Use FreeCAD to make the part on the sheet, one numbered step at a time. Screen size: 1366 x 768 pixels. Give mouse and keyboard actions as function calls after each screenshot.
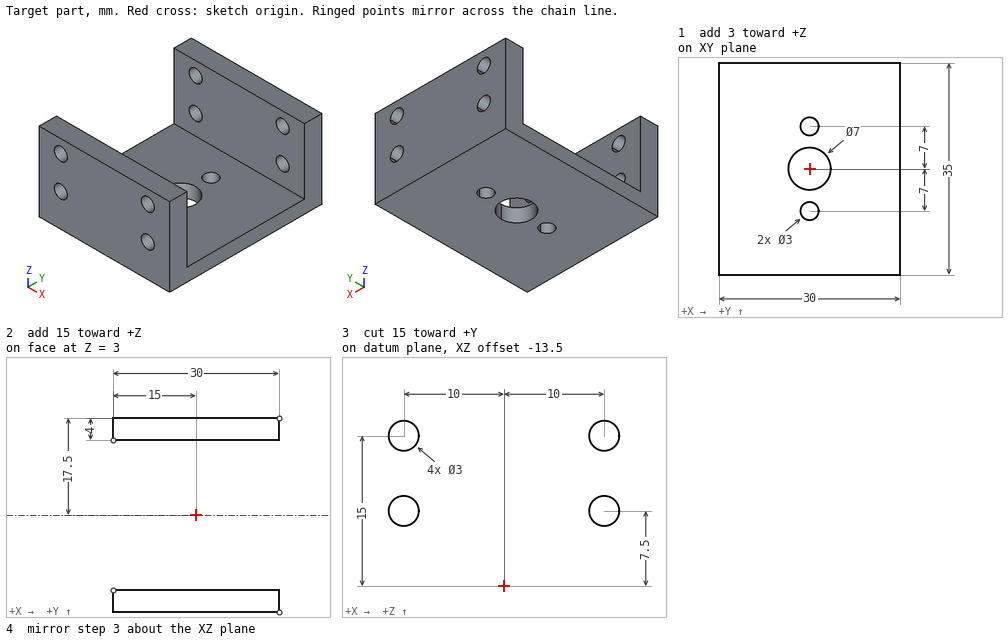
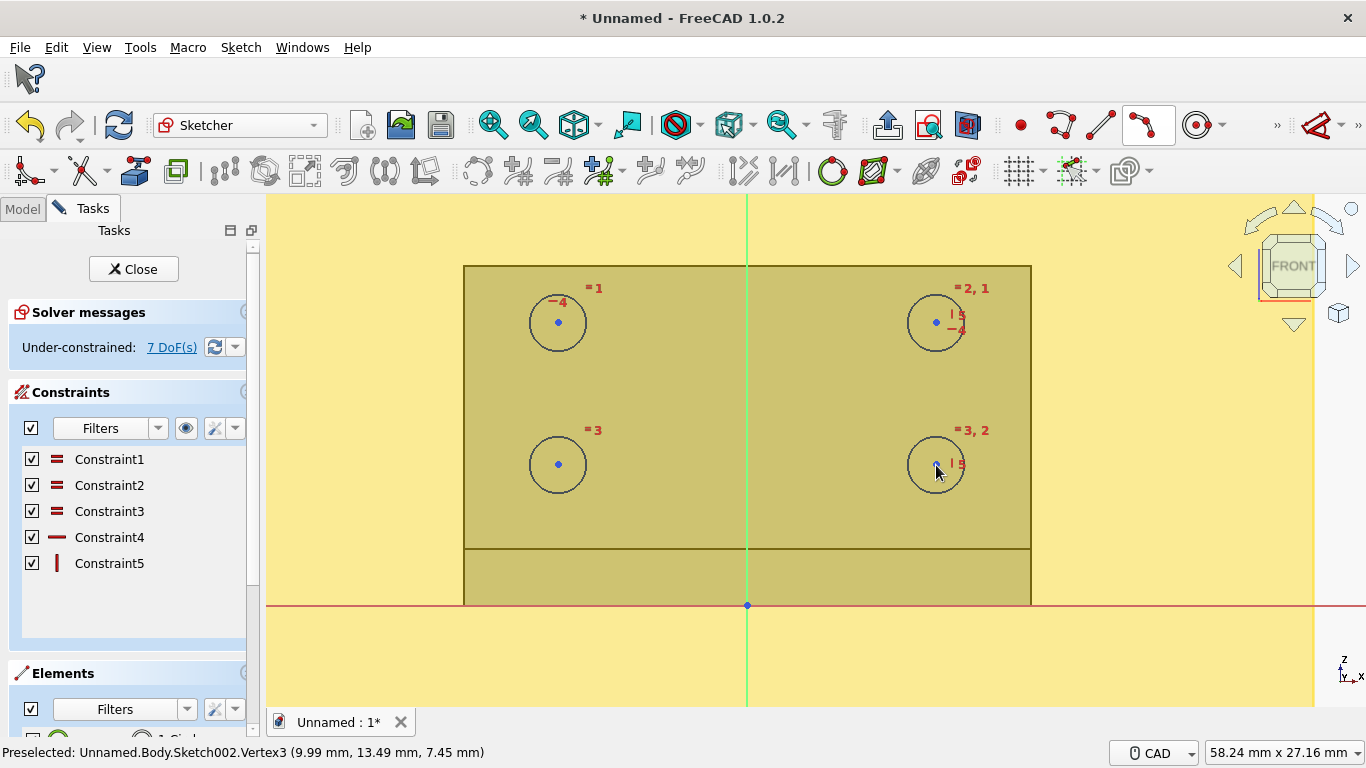
click(558, 323)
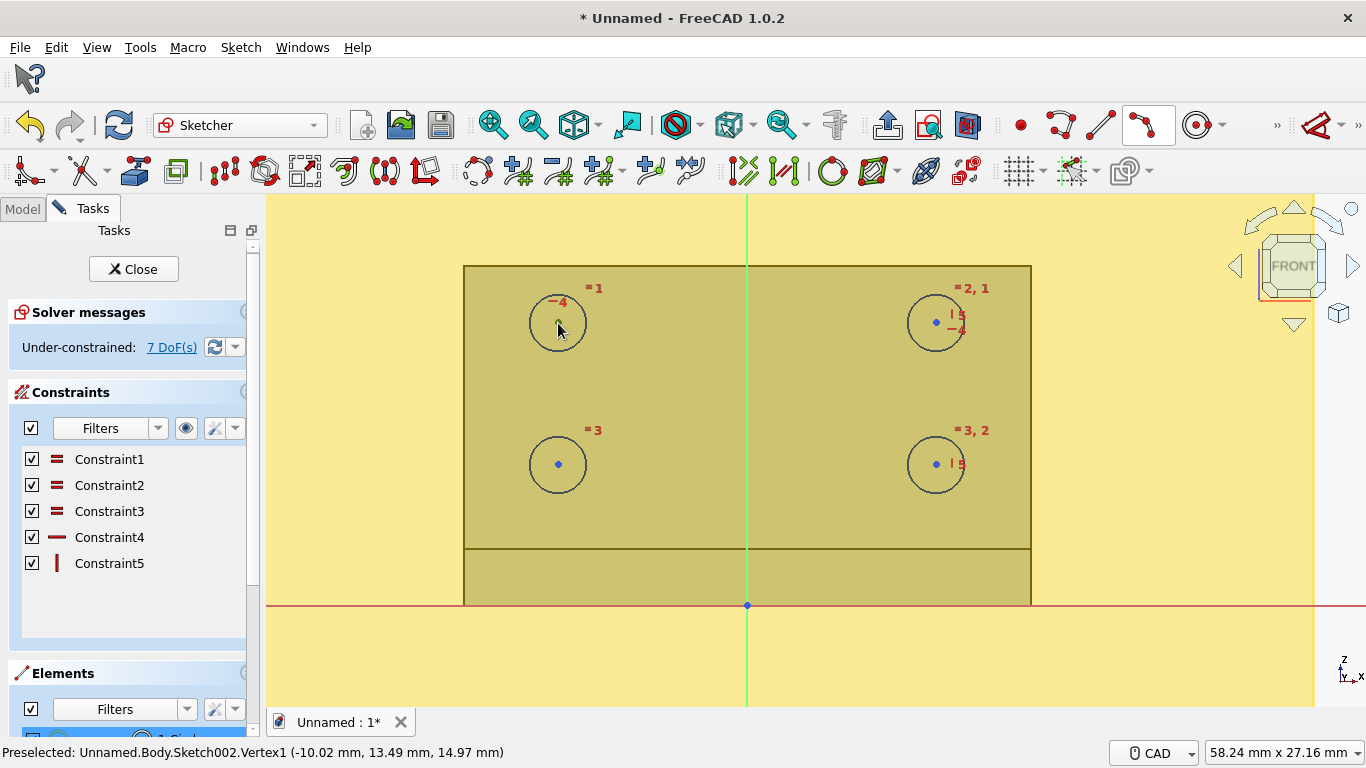
click(558, 465)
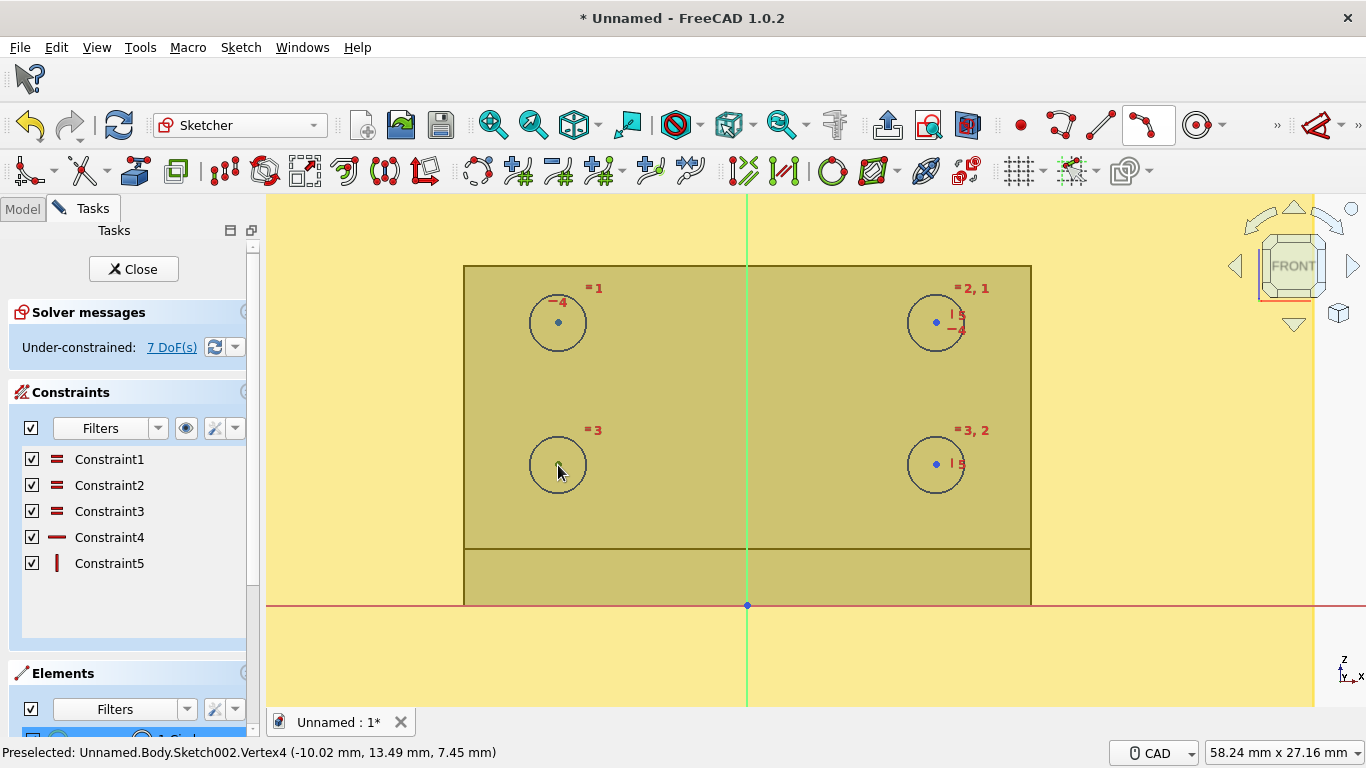
key(v)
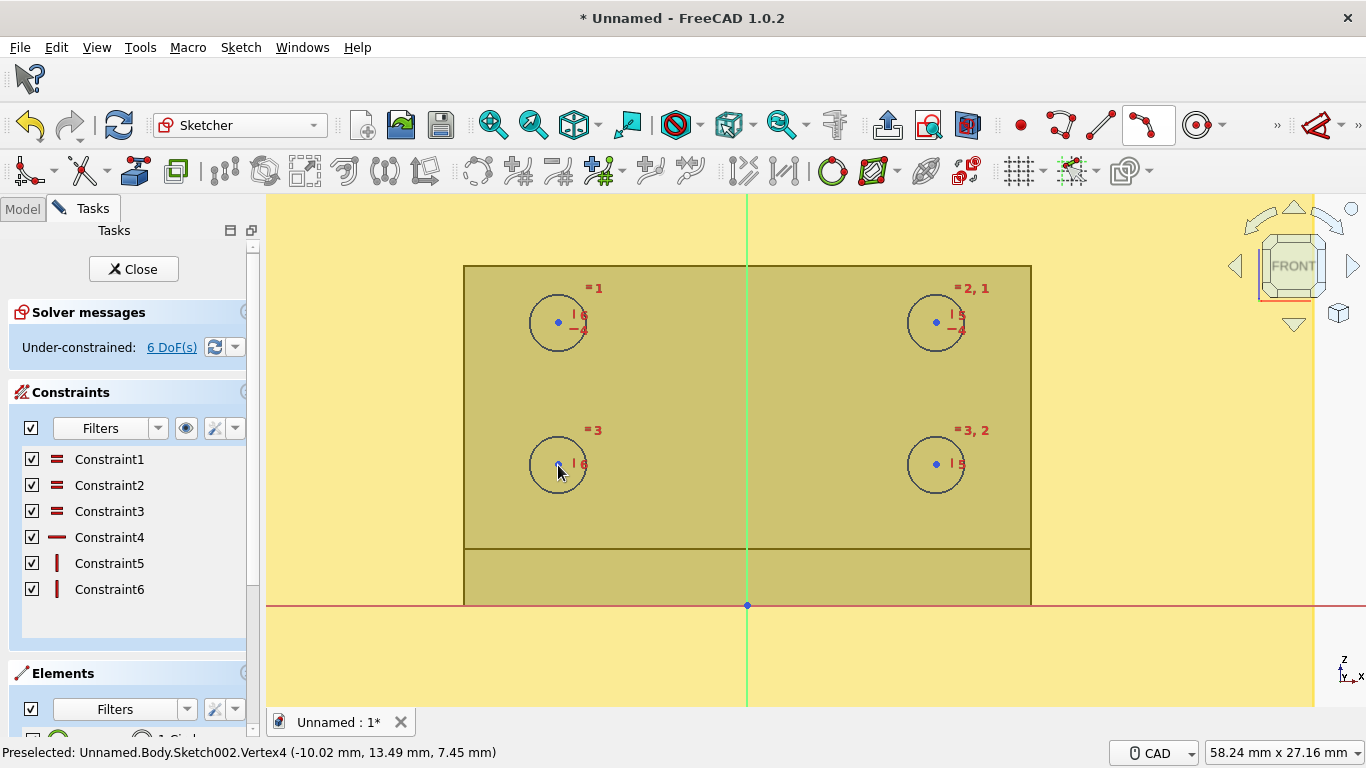
click(936, 465)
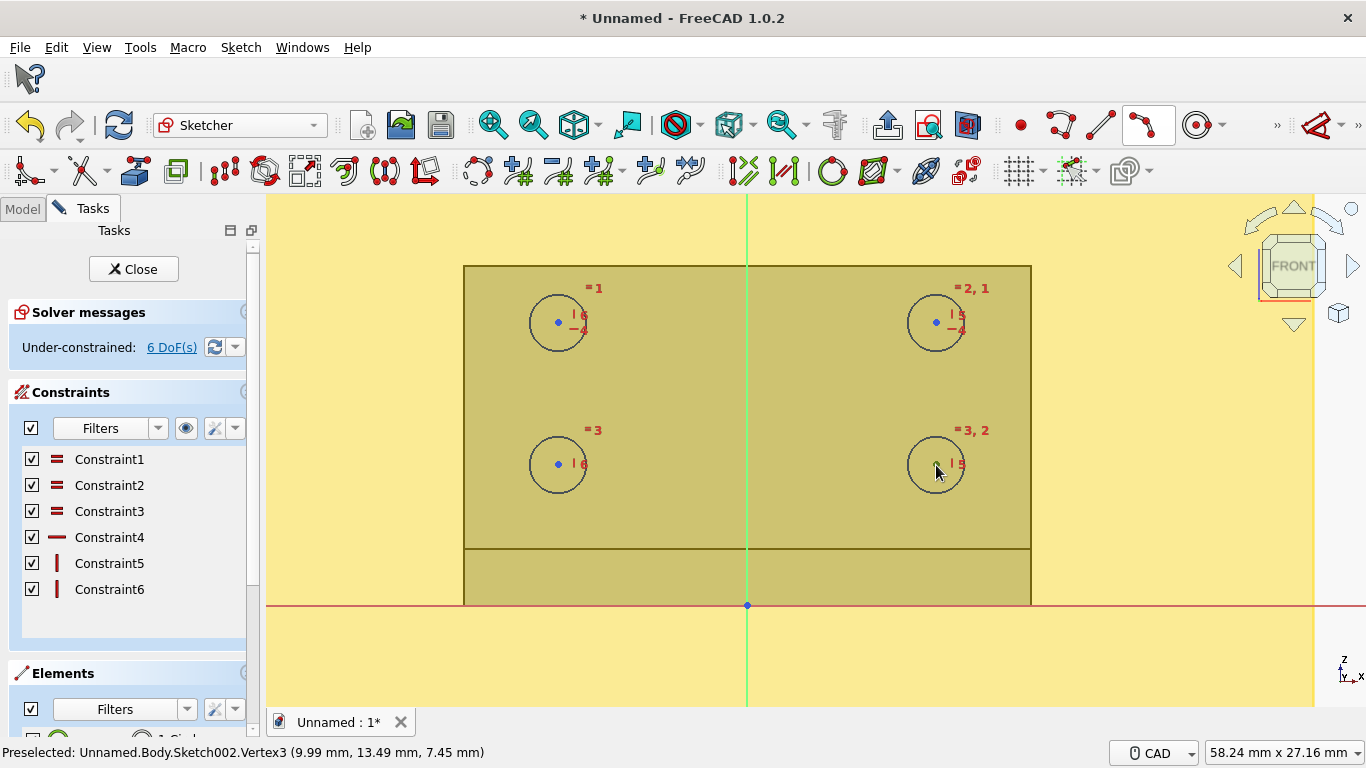
click(558, 465)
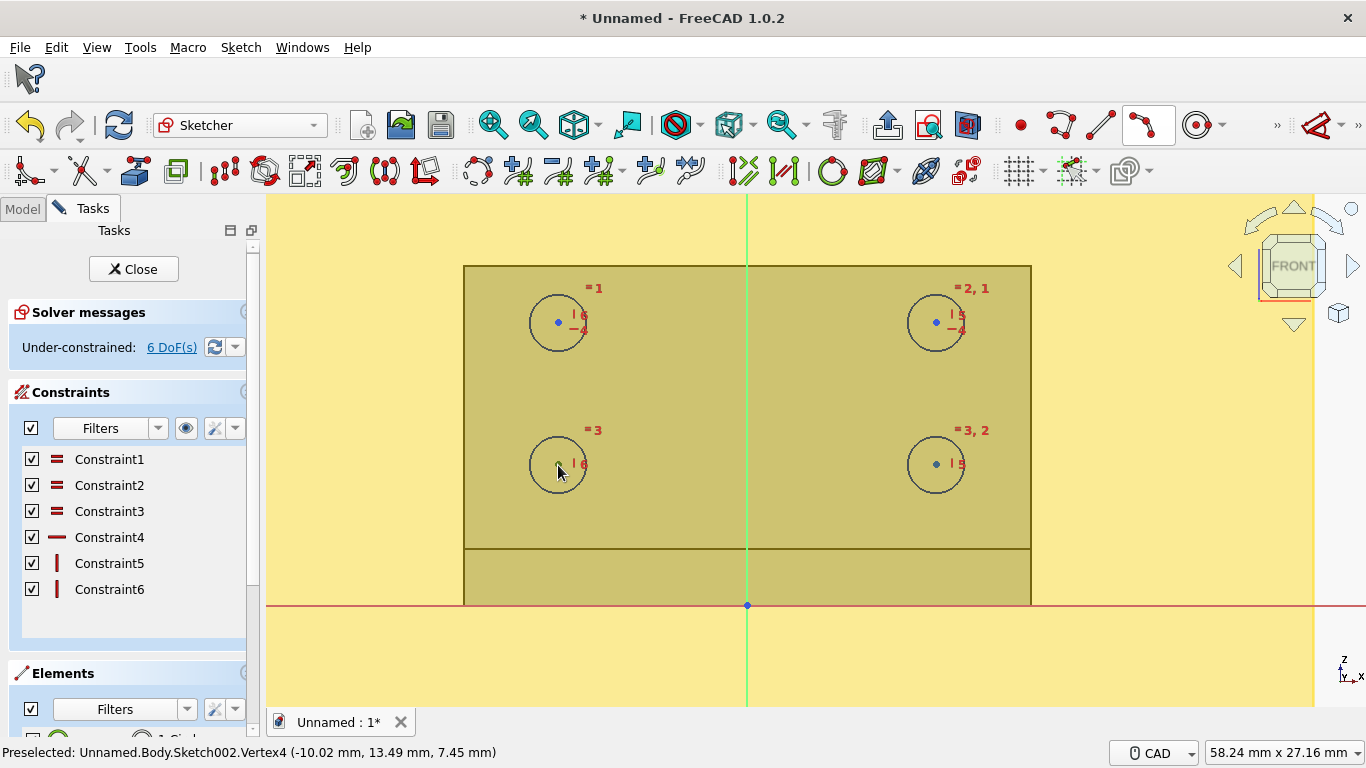
key(h)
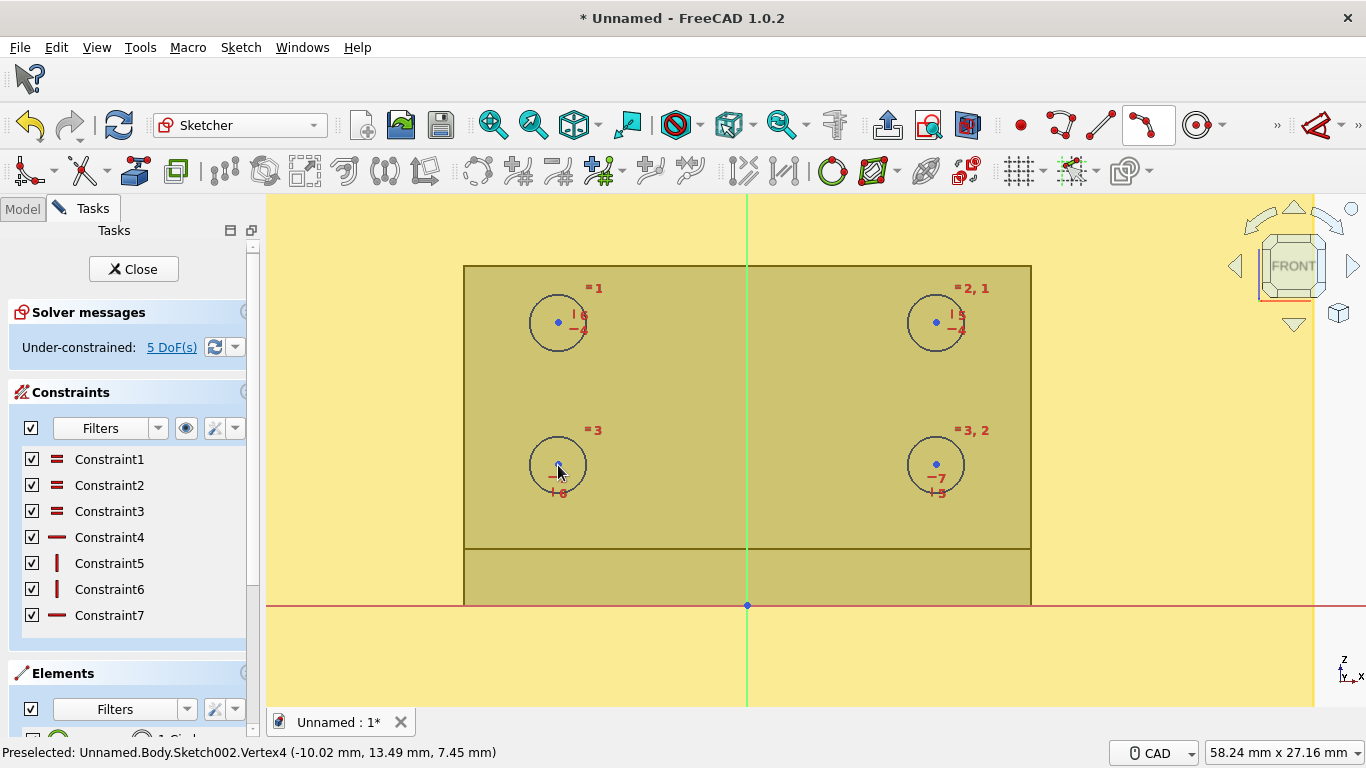
click(1316, 126)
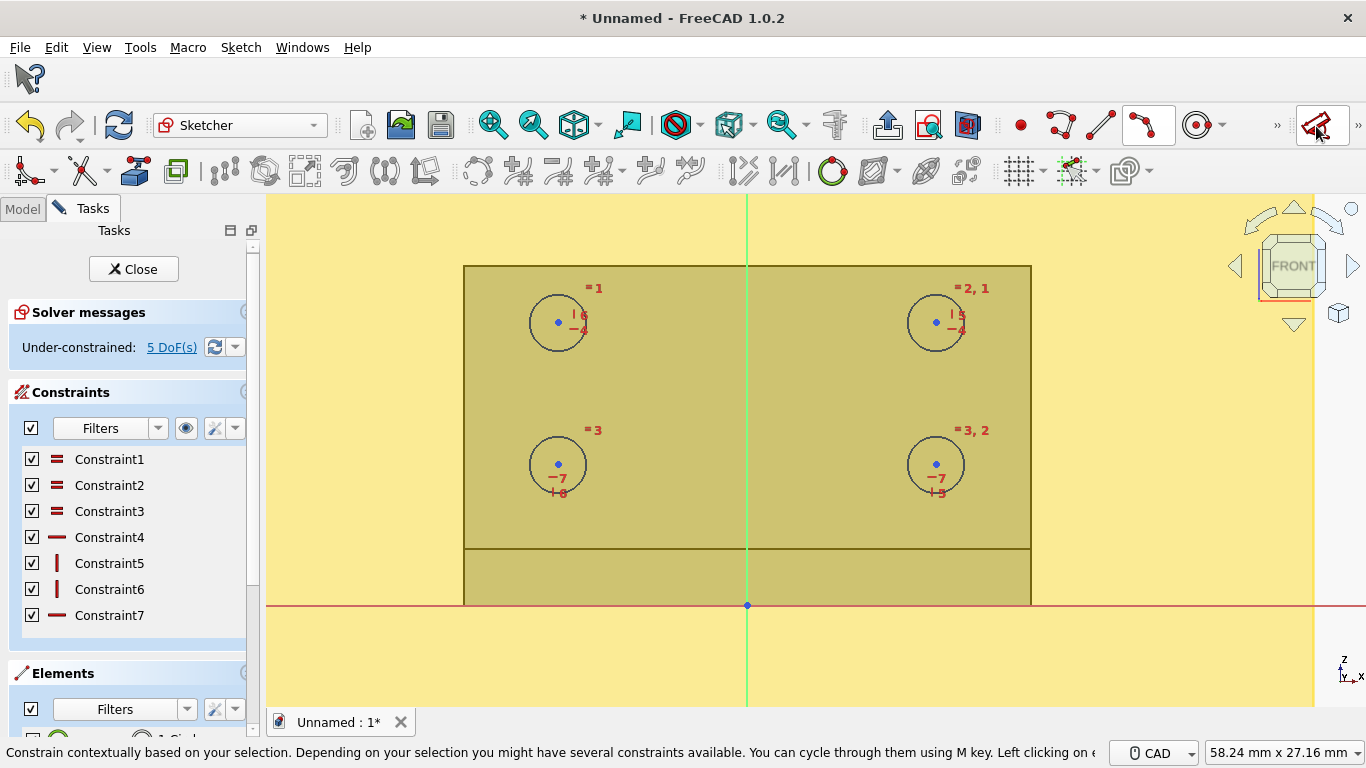
click(578, 303)
click(601, 280)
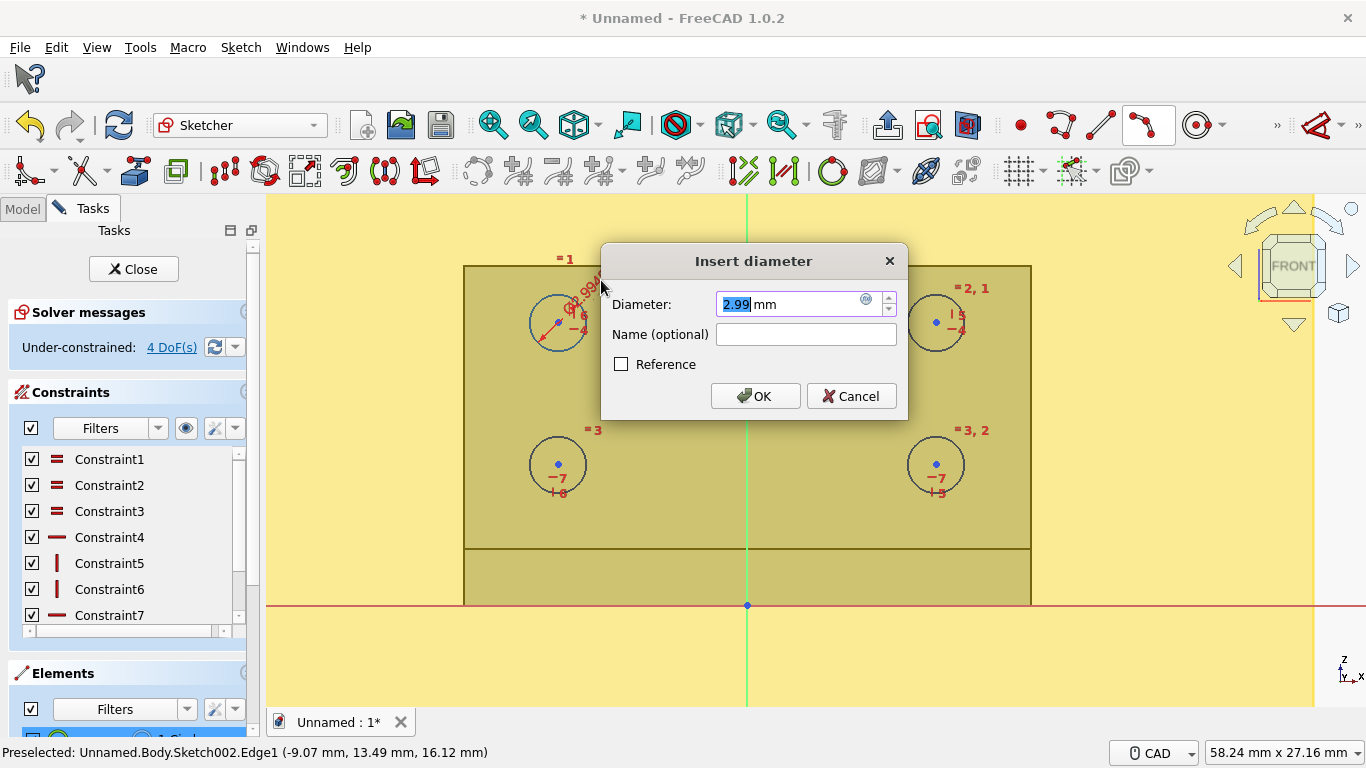
text(3)
key(Return)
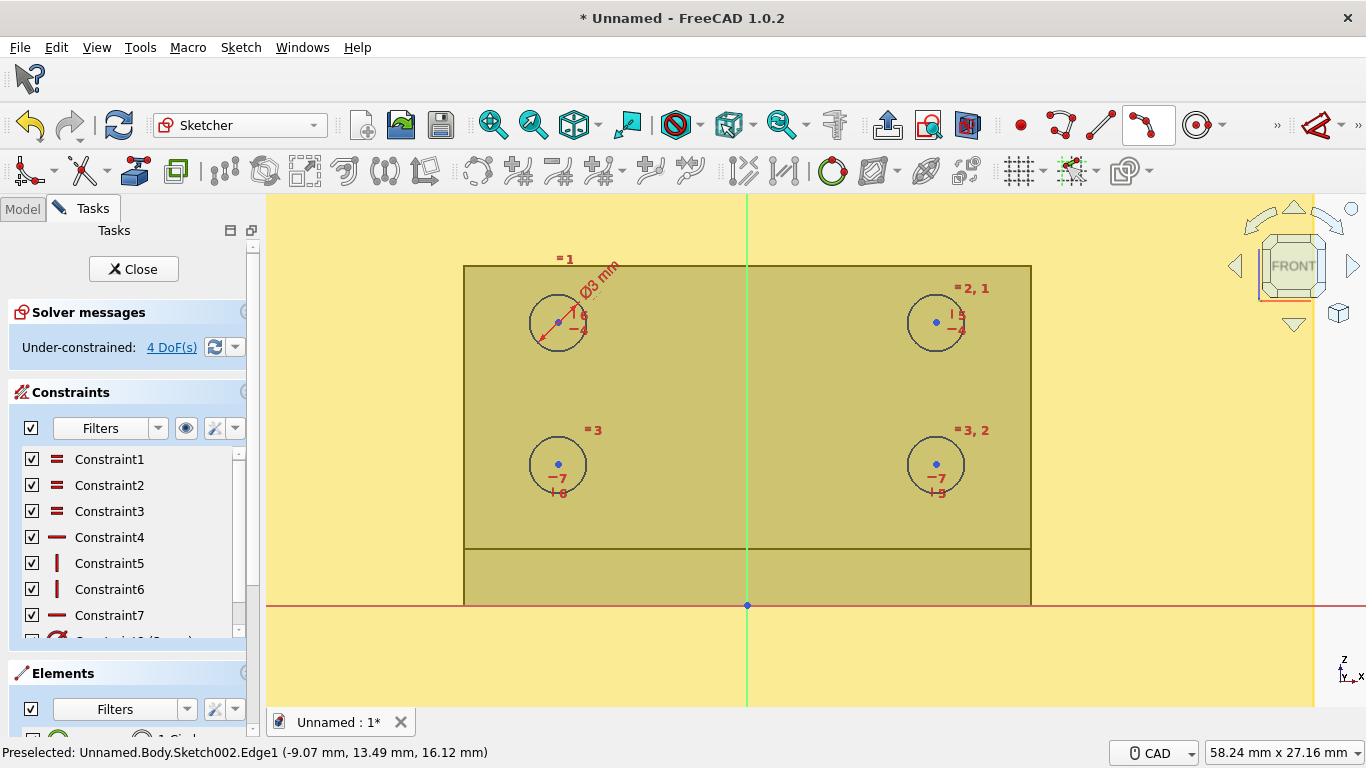
click(558, 323)
click(653, 640)